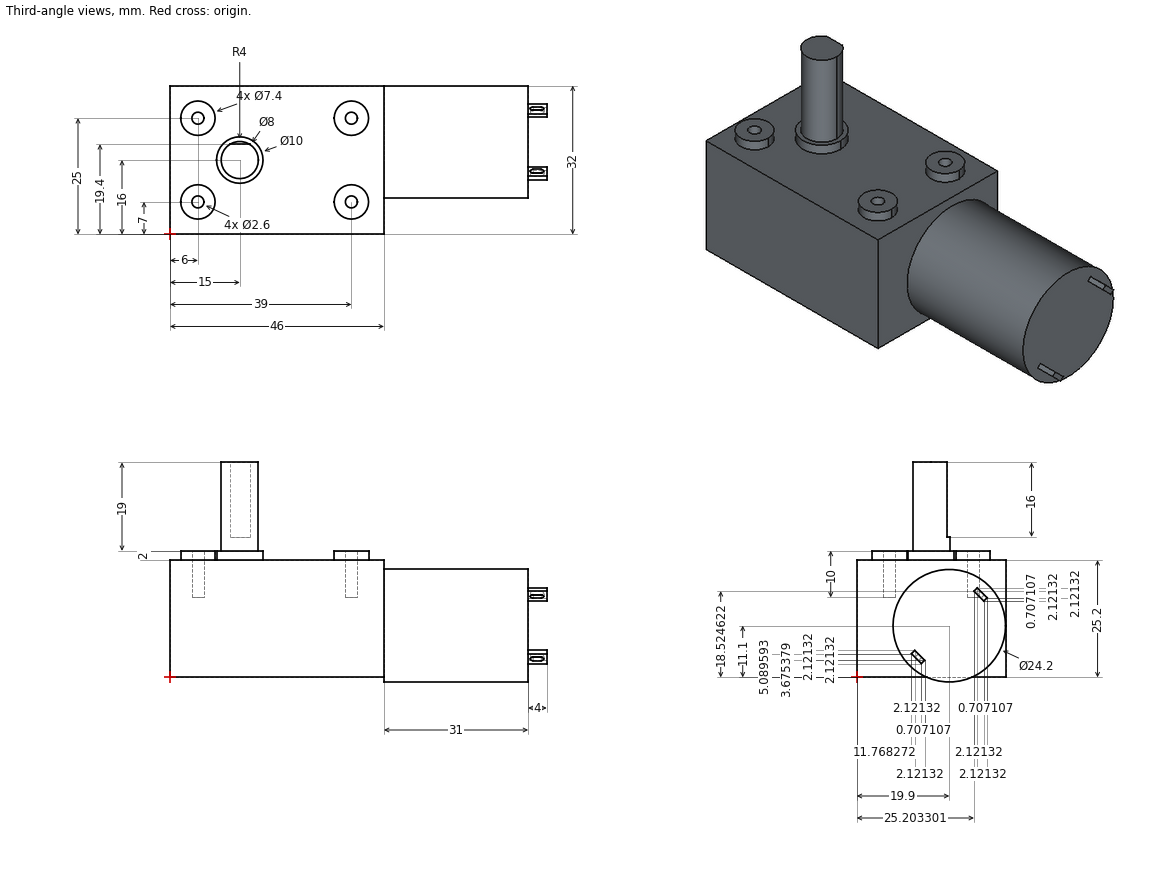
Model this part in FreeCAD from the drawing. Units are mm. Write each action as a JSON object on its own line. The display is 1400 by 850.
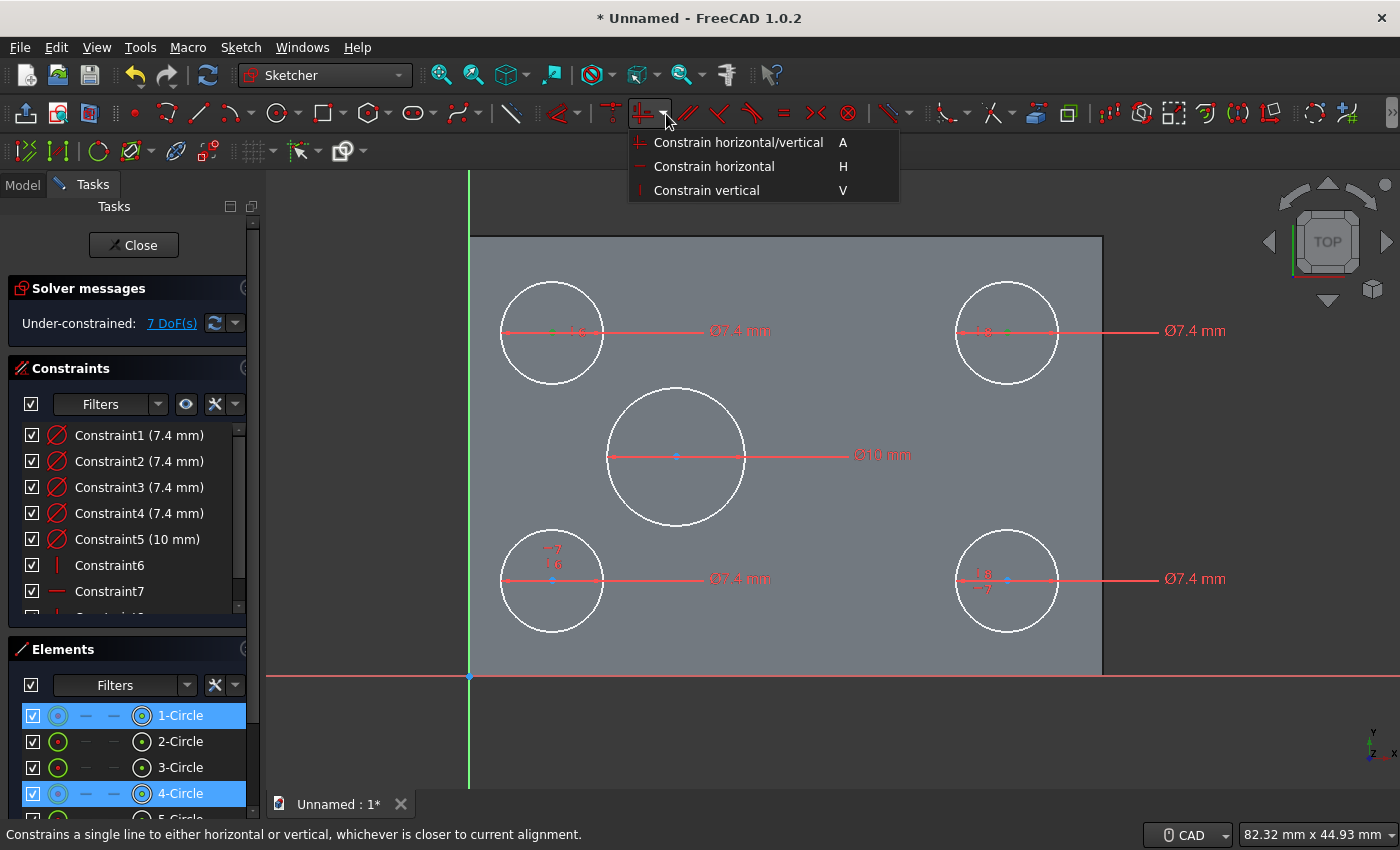
{"action": "left_click", "coordinate": [764, 166]}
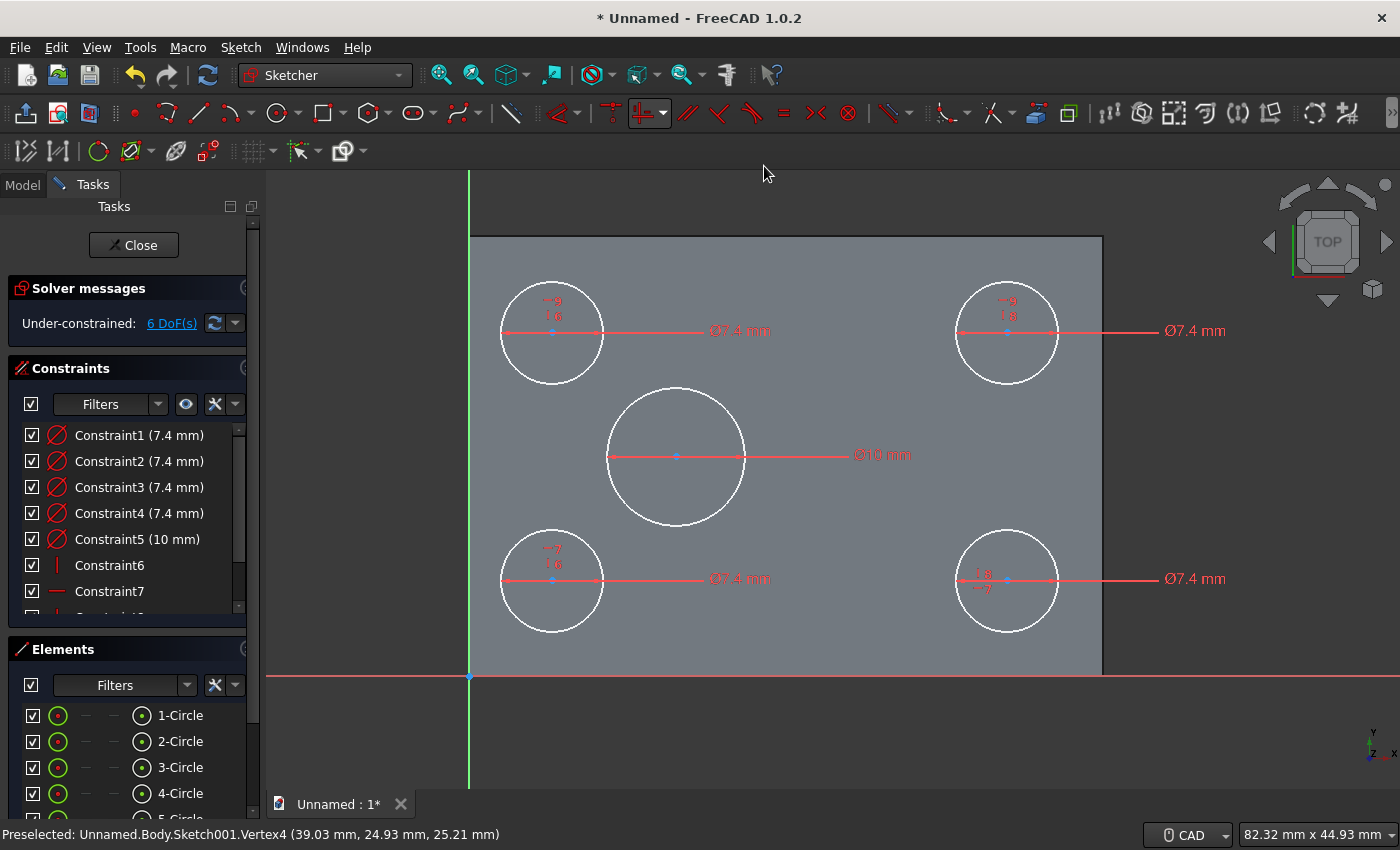
{"action": "left_click", "coordinate": [558, 114]}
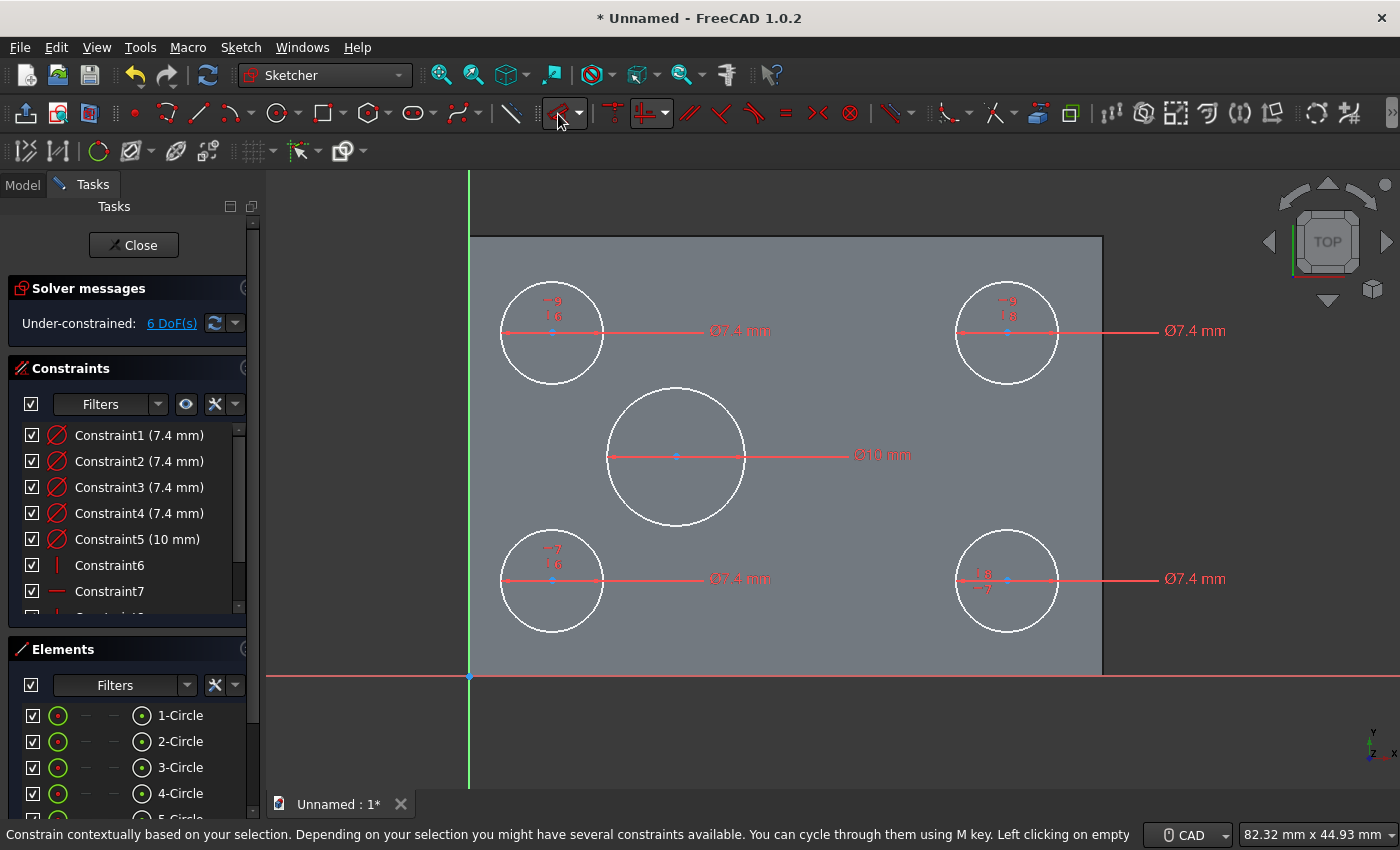
{"action": "left_click", "coordinate": [552, 333]}
{"action": "left_click", "coordinate": [511, 710]}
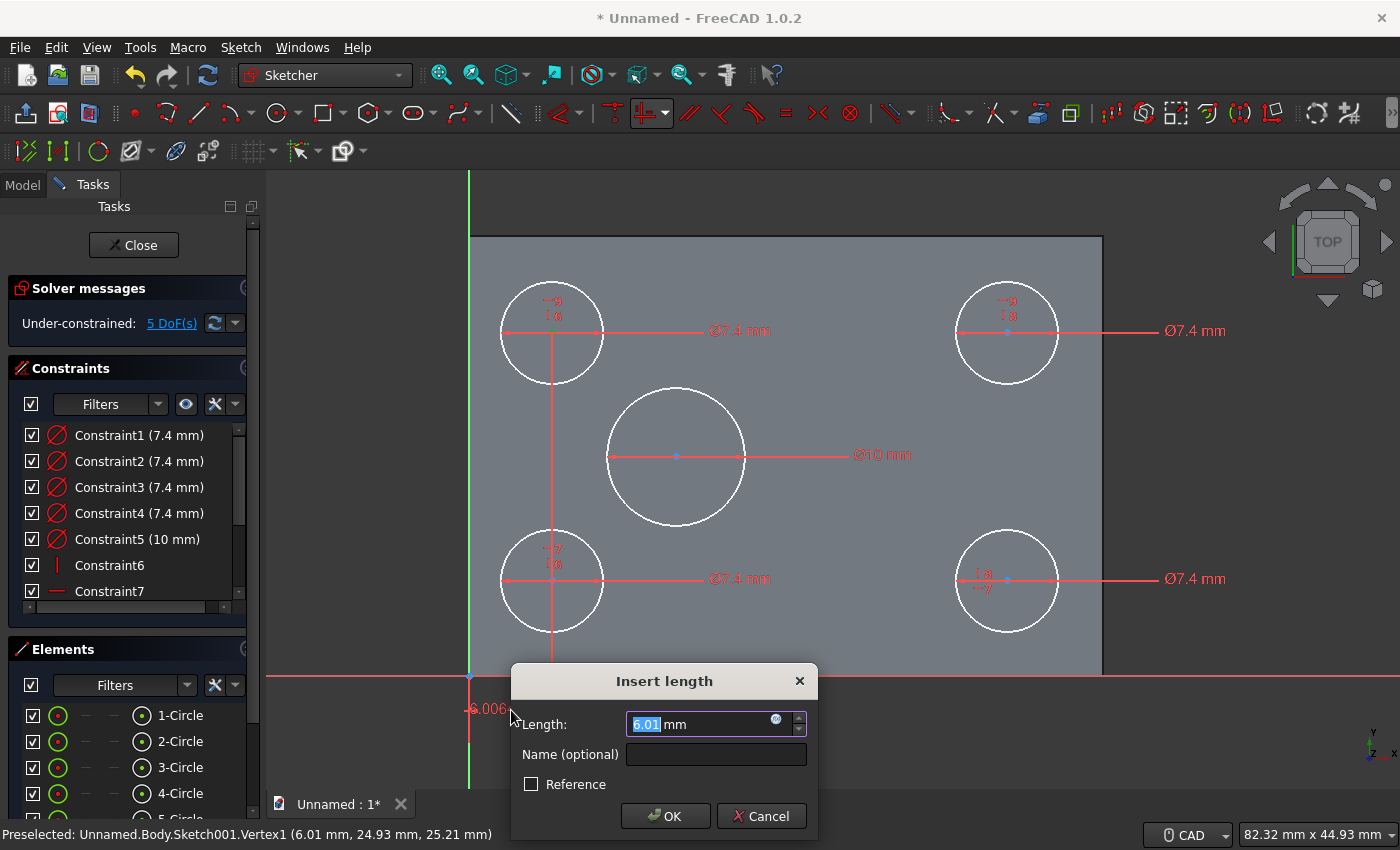
{"action": "type", "text": "6"}
{"action": "key", "text": "Return"}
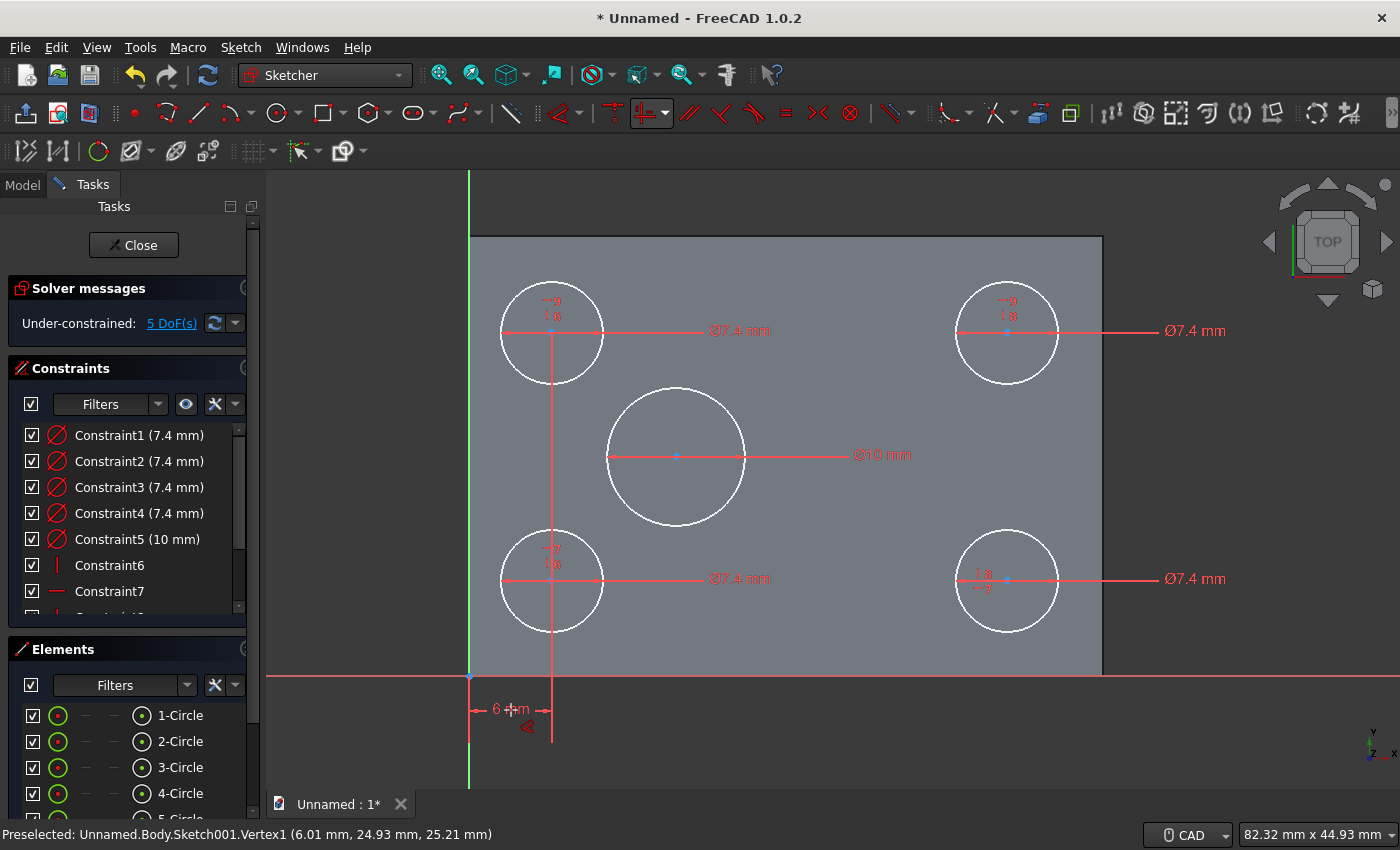
{"action": "left_click", "coordinate": [552, 581]}
{"action": "left_click", "coordinate": [435, 629]}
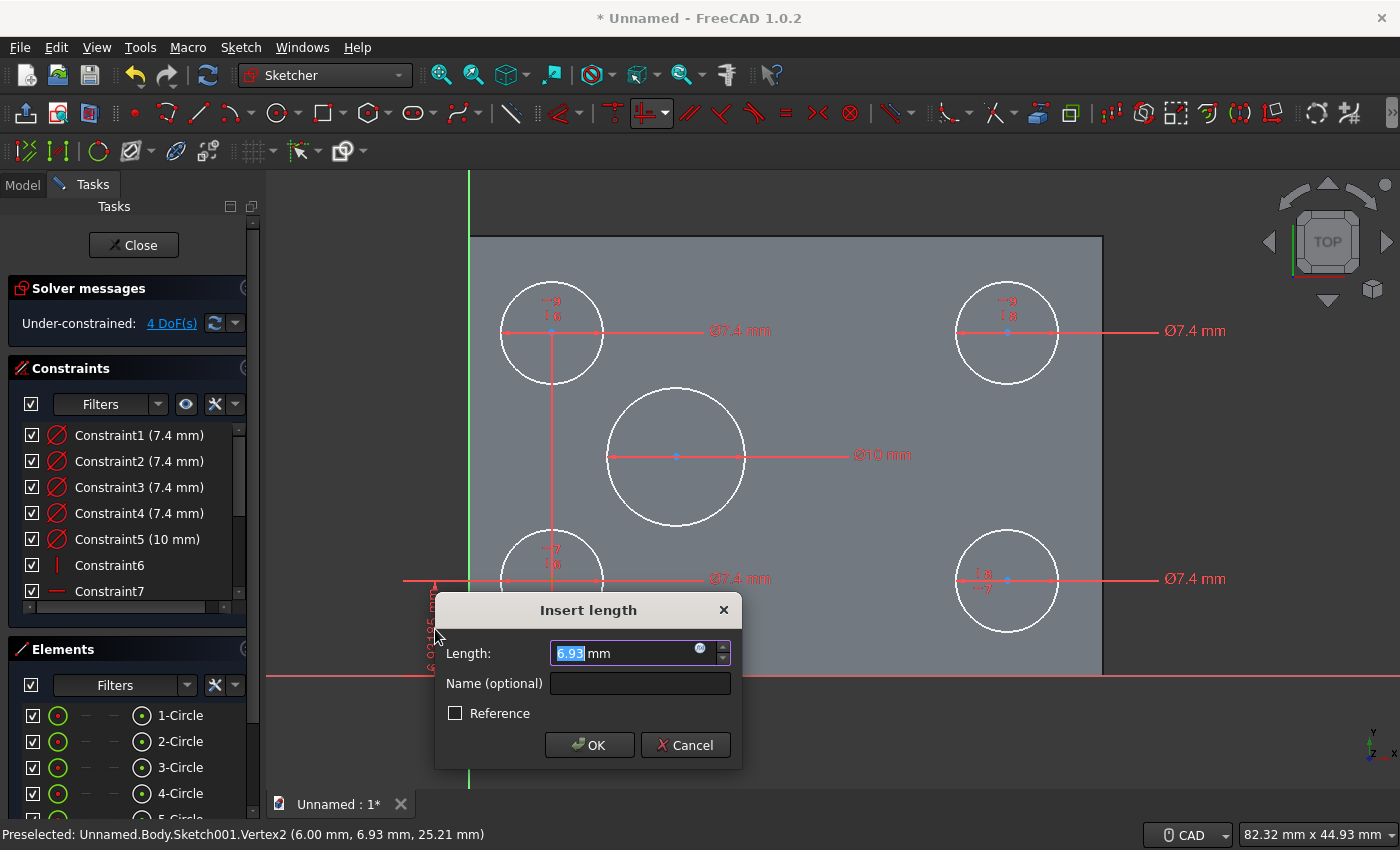
{"action": "type", "text": "7"}
{"action": "key", "text": "Return"}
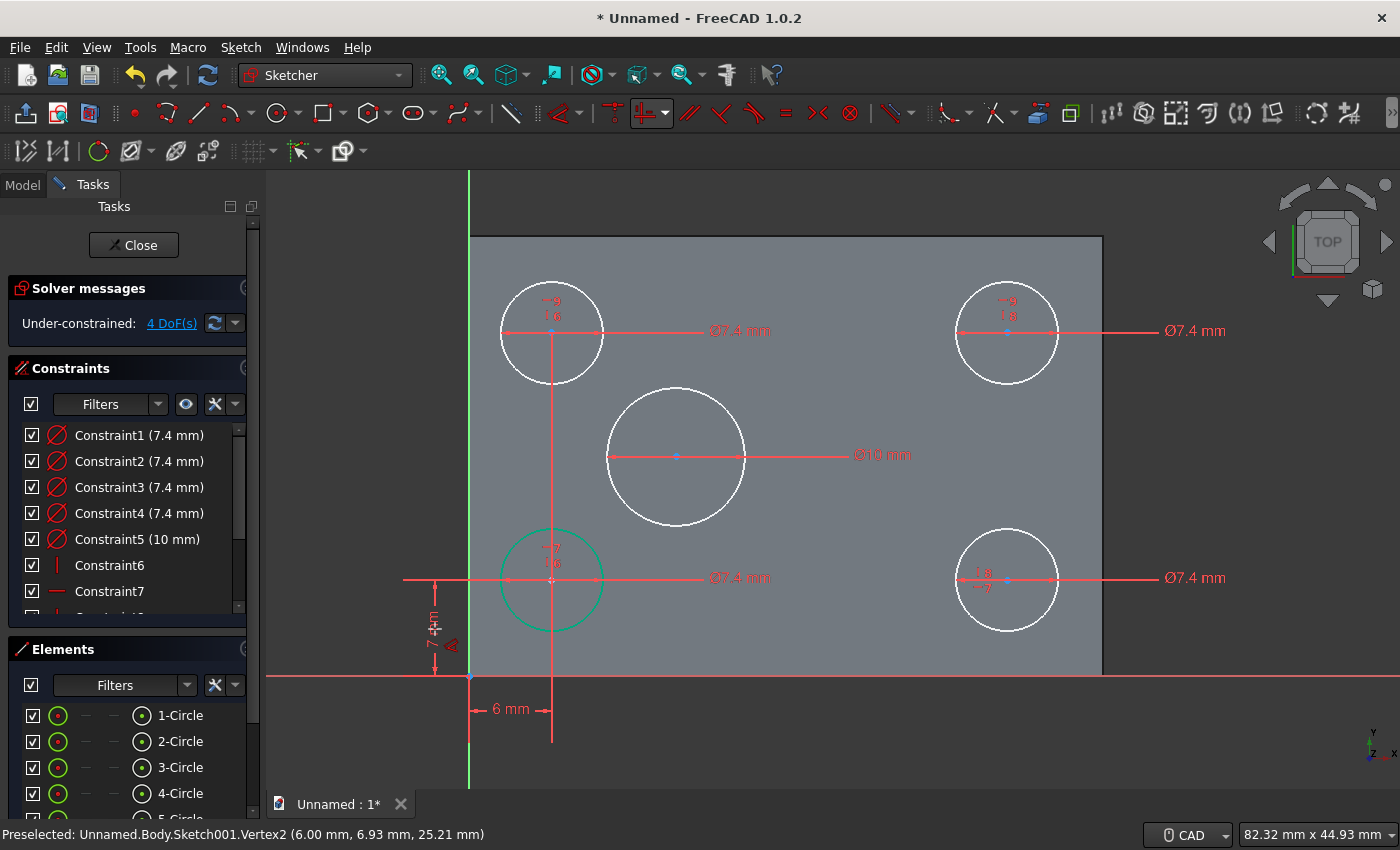
{"action": "left_click", "coordinate": [552, 333]}
{"action": "left_click", "coordinate": [435, 505]}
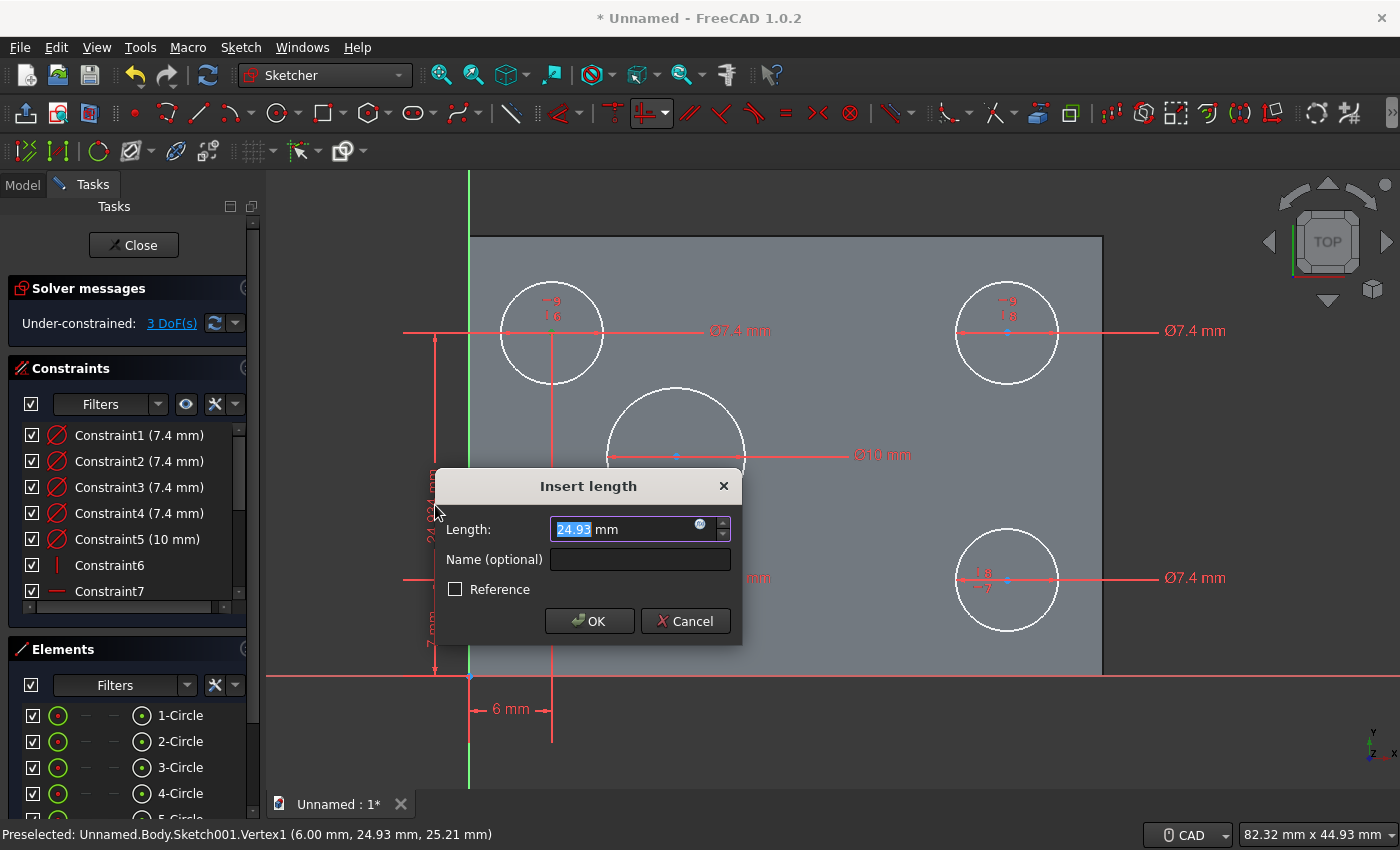
{"action": "type", "text": "25"}
{"action": "key", "text": "Return"}